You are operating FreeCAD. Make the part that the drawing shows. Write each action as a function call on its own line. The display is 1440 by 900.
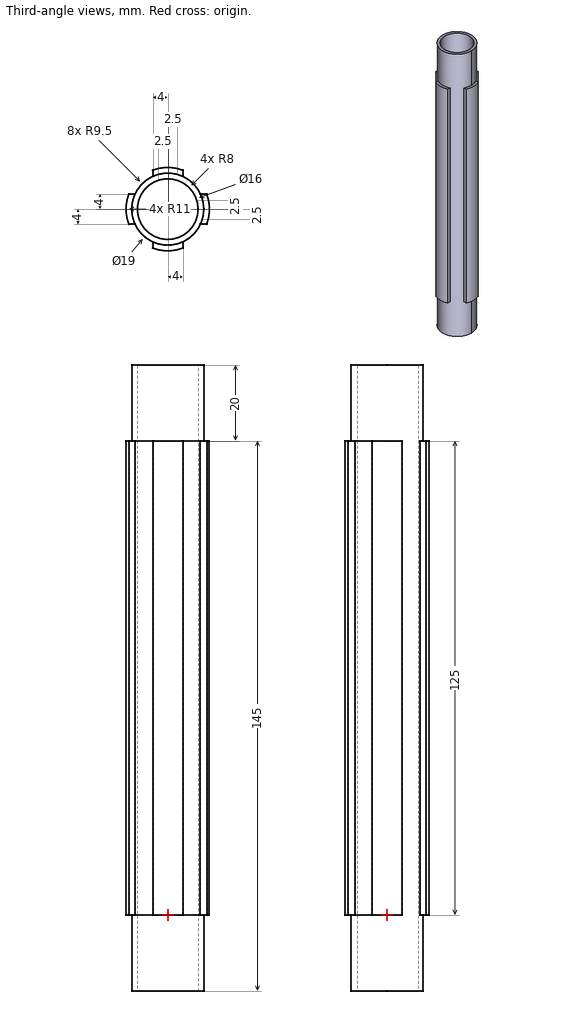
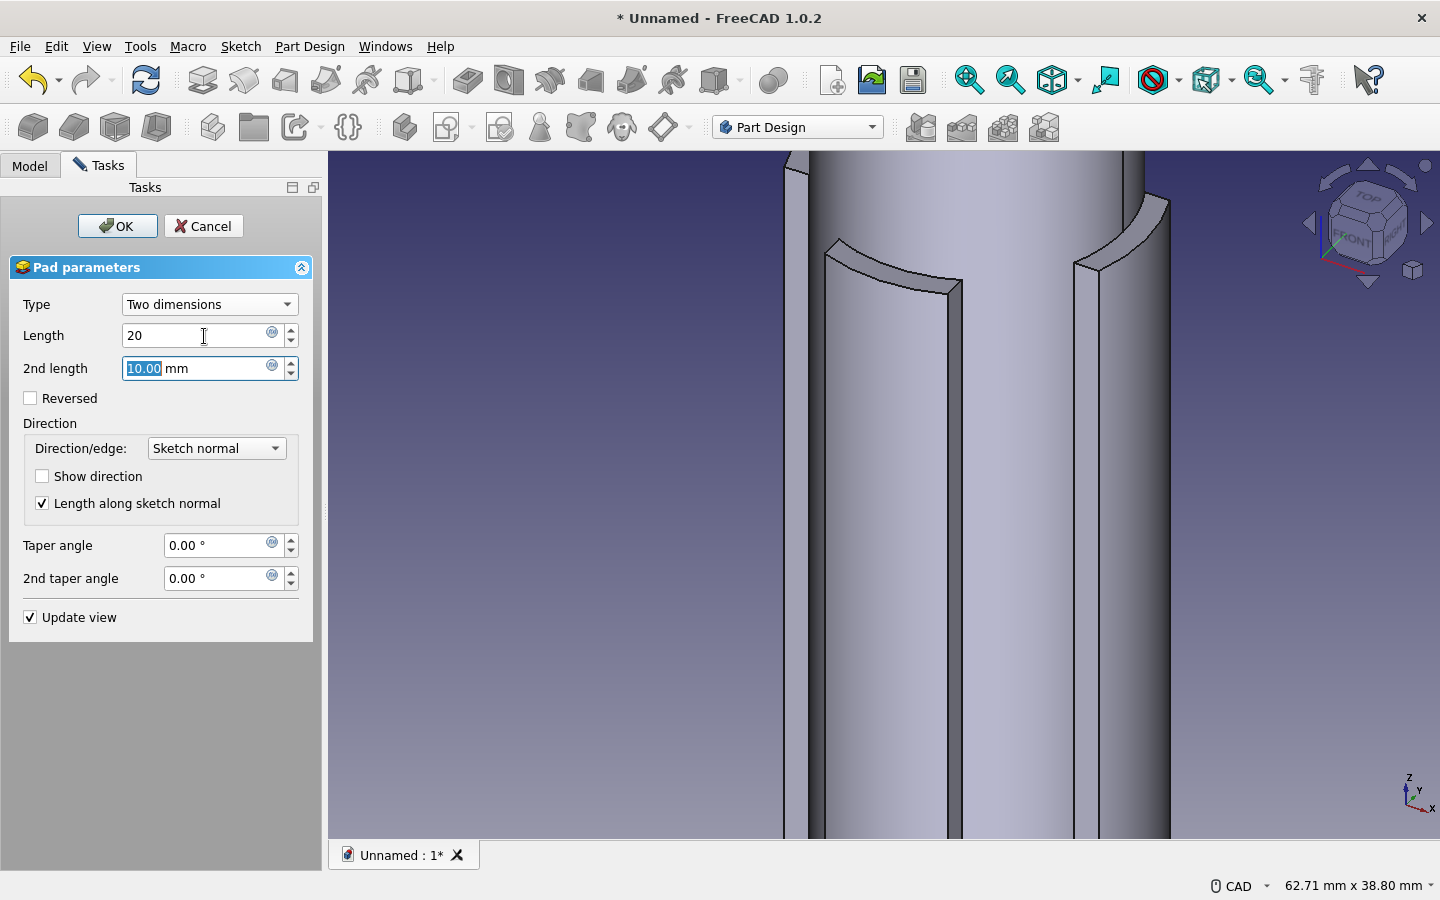
text(145)
key(Tab)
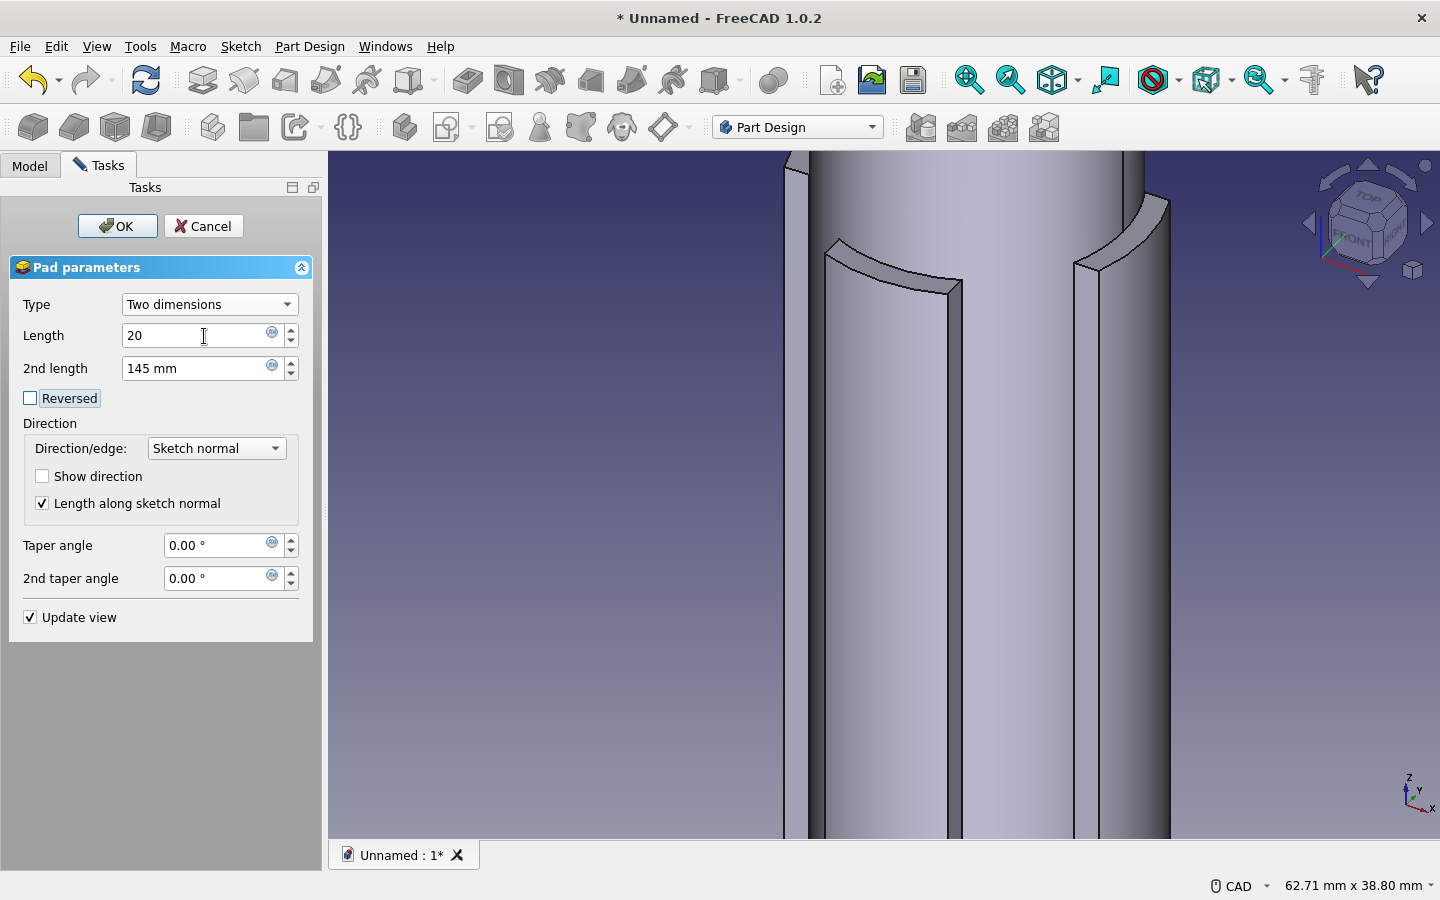
click(118, 226)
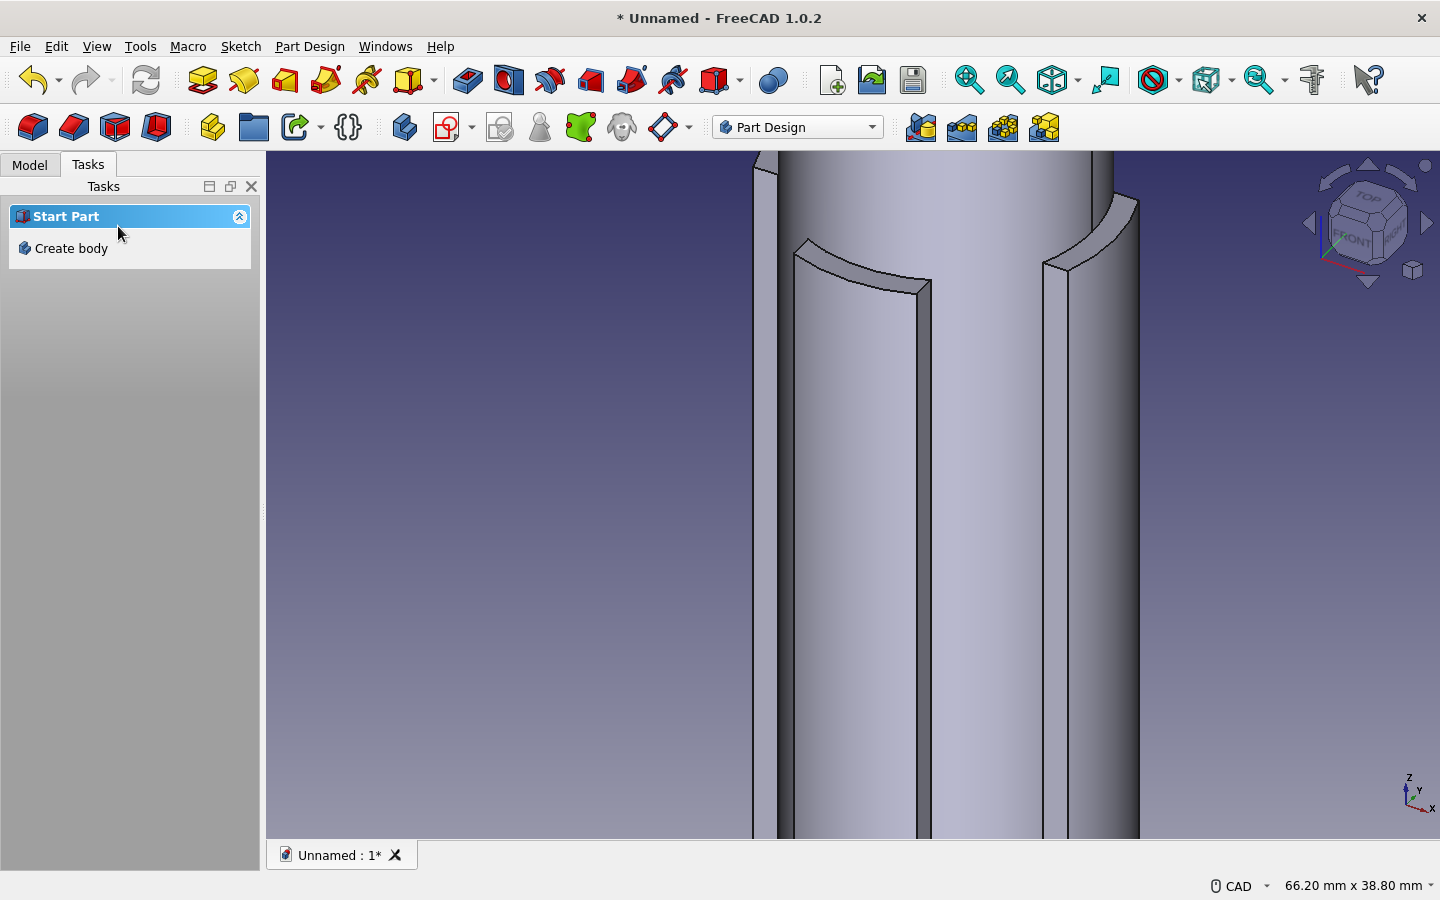
key(0)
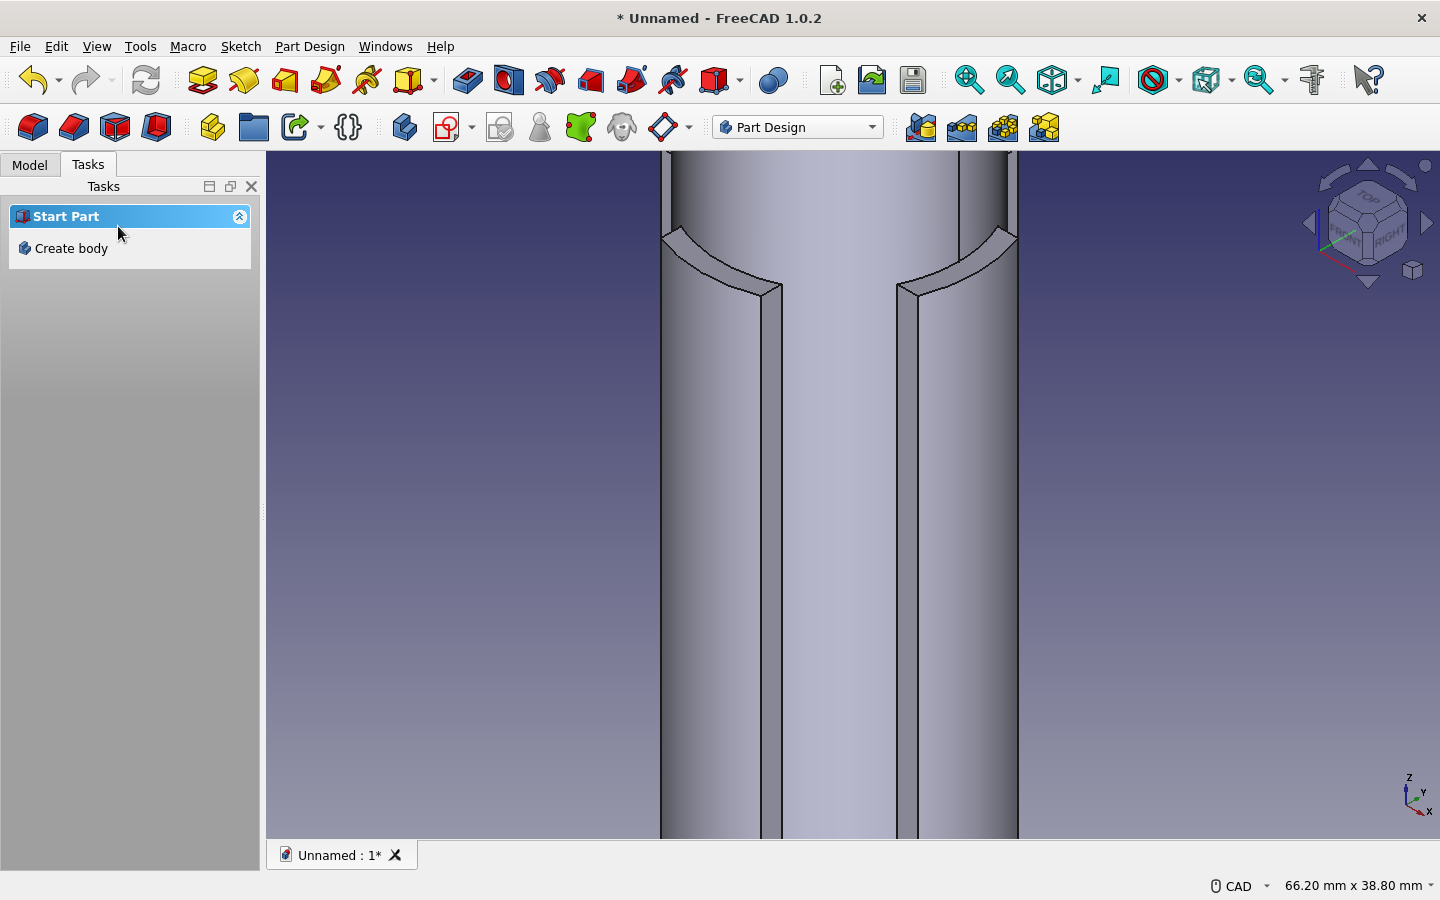
click(970, 80)